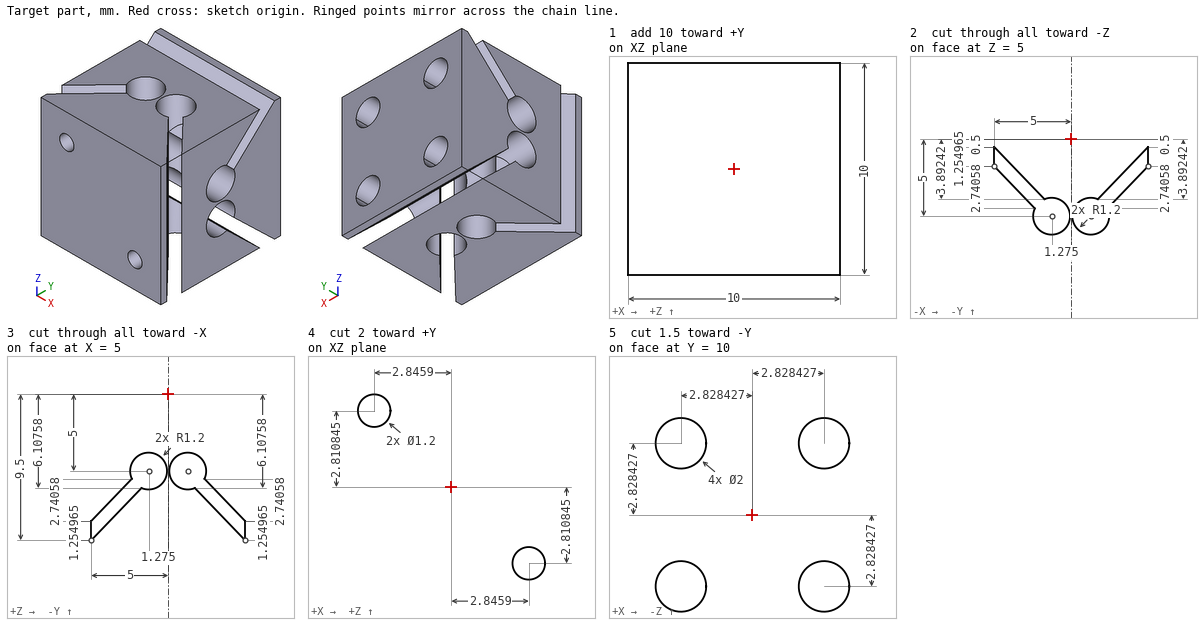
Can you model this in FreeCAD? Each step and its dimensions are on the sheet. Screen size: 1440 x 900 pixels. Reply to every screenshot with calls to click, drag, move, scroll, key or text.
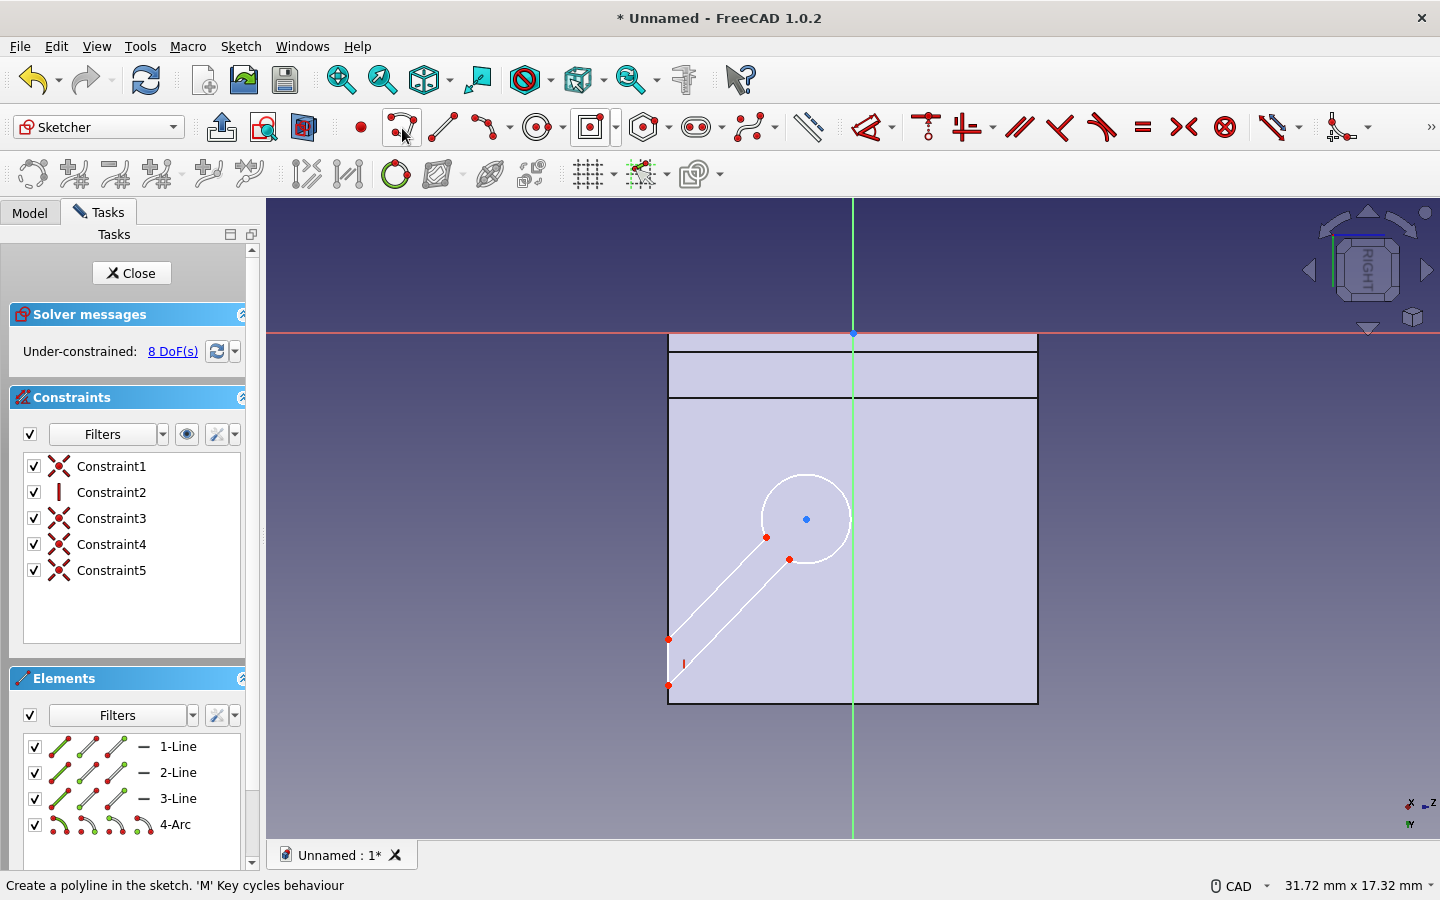
click(917, 559)
click(1038, 685)
click(1038, 639)
click(940, 537)
right_click(940, 537)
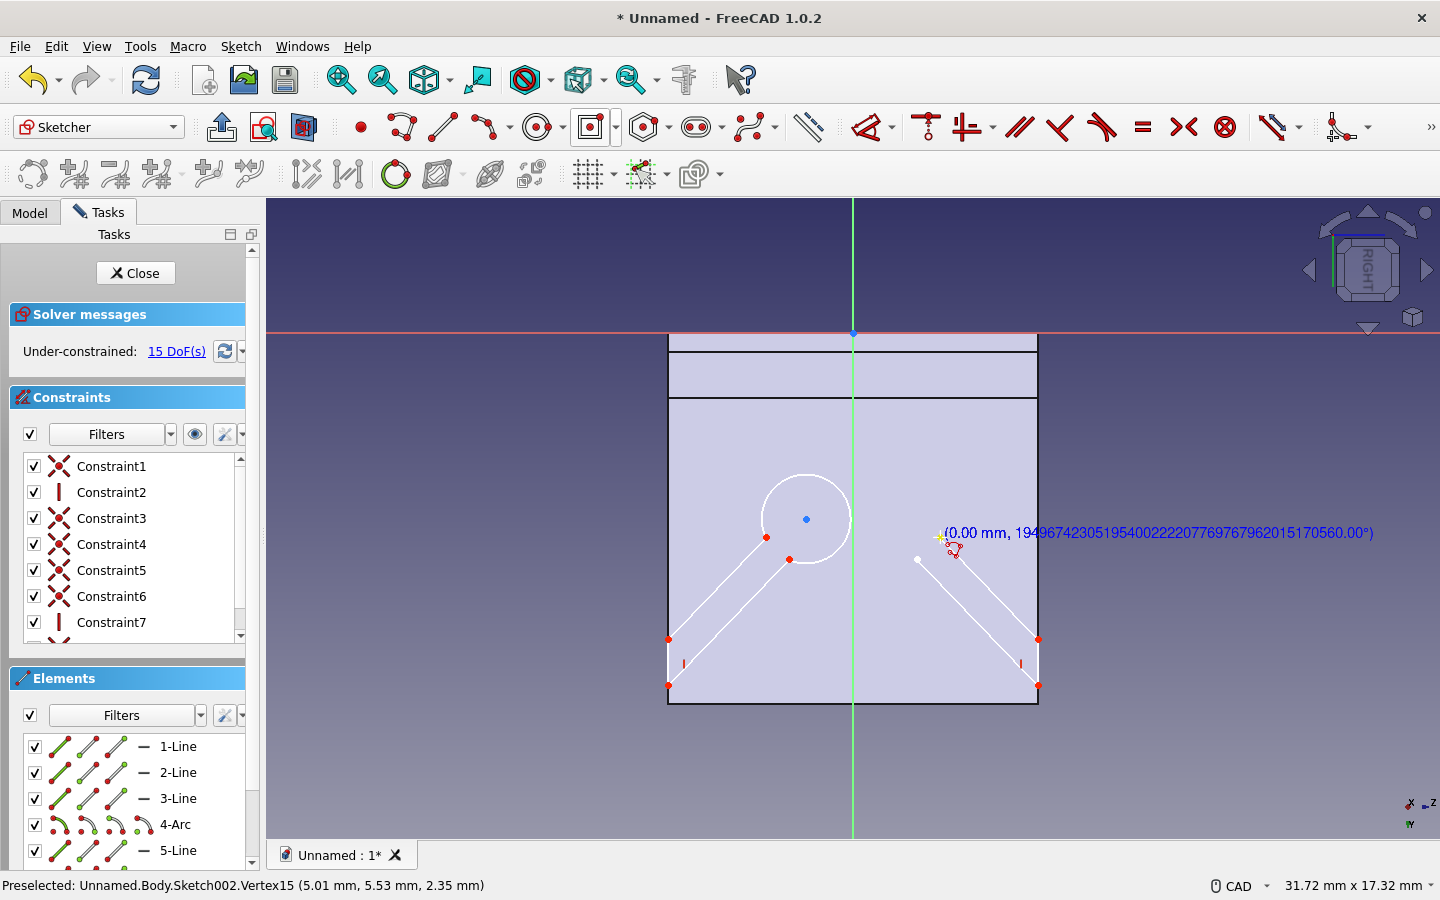
key(g)
key(3)
key(a)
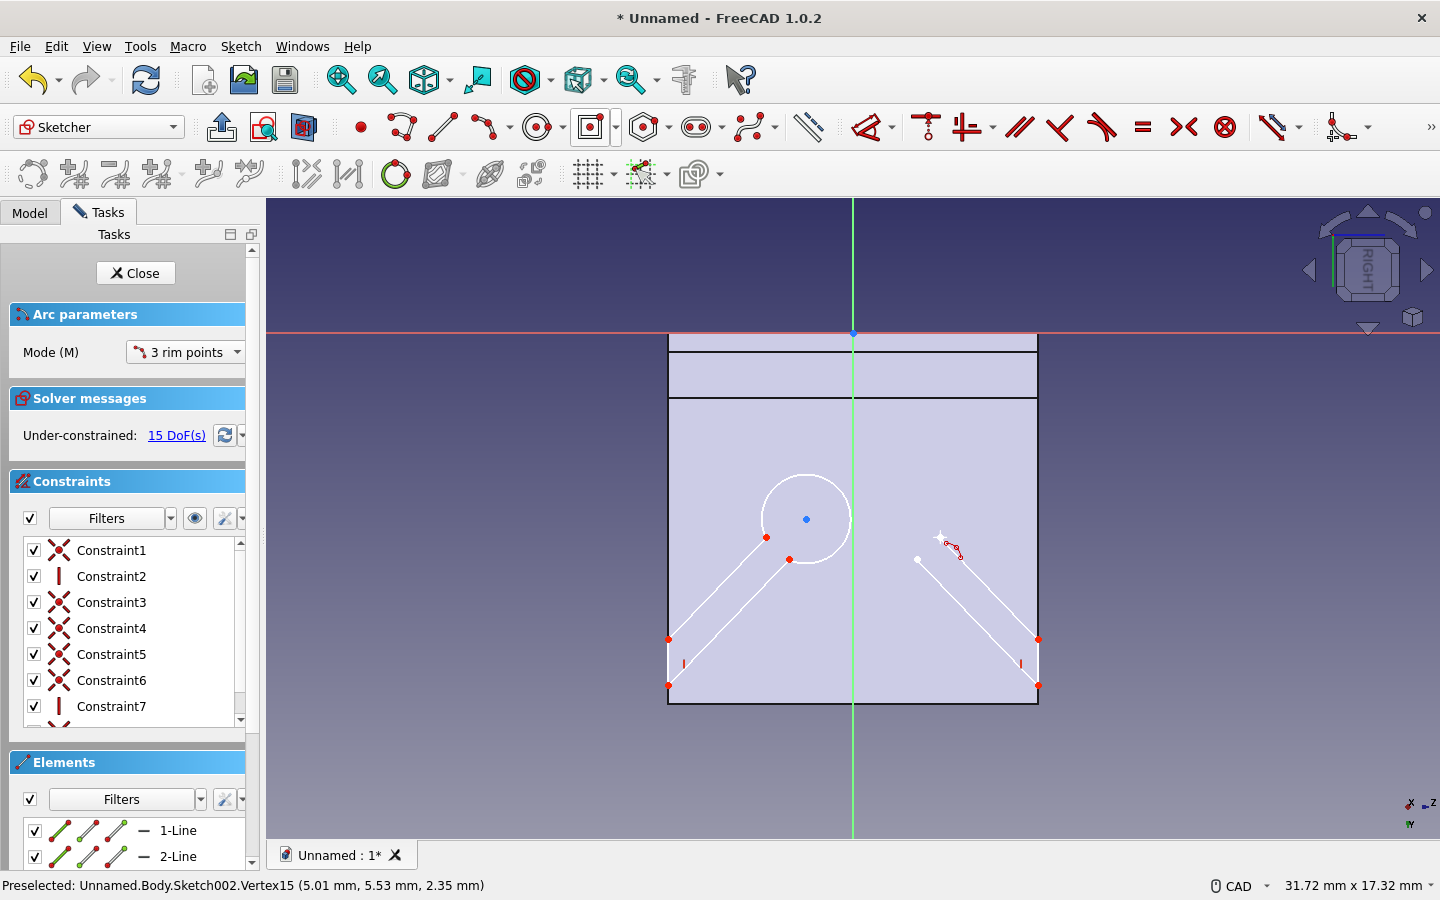
click(940, 538)
click(917, 560)
click(869, 486)
key(Escape)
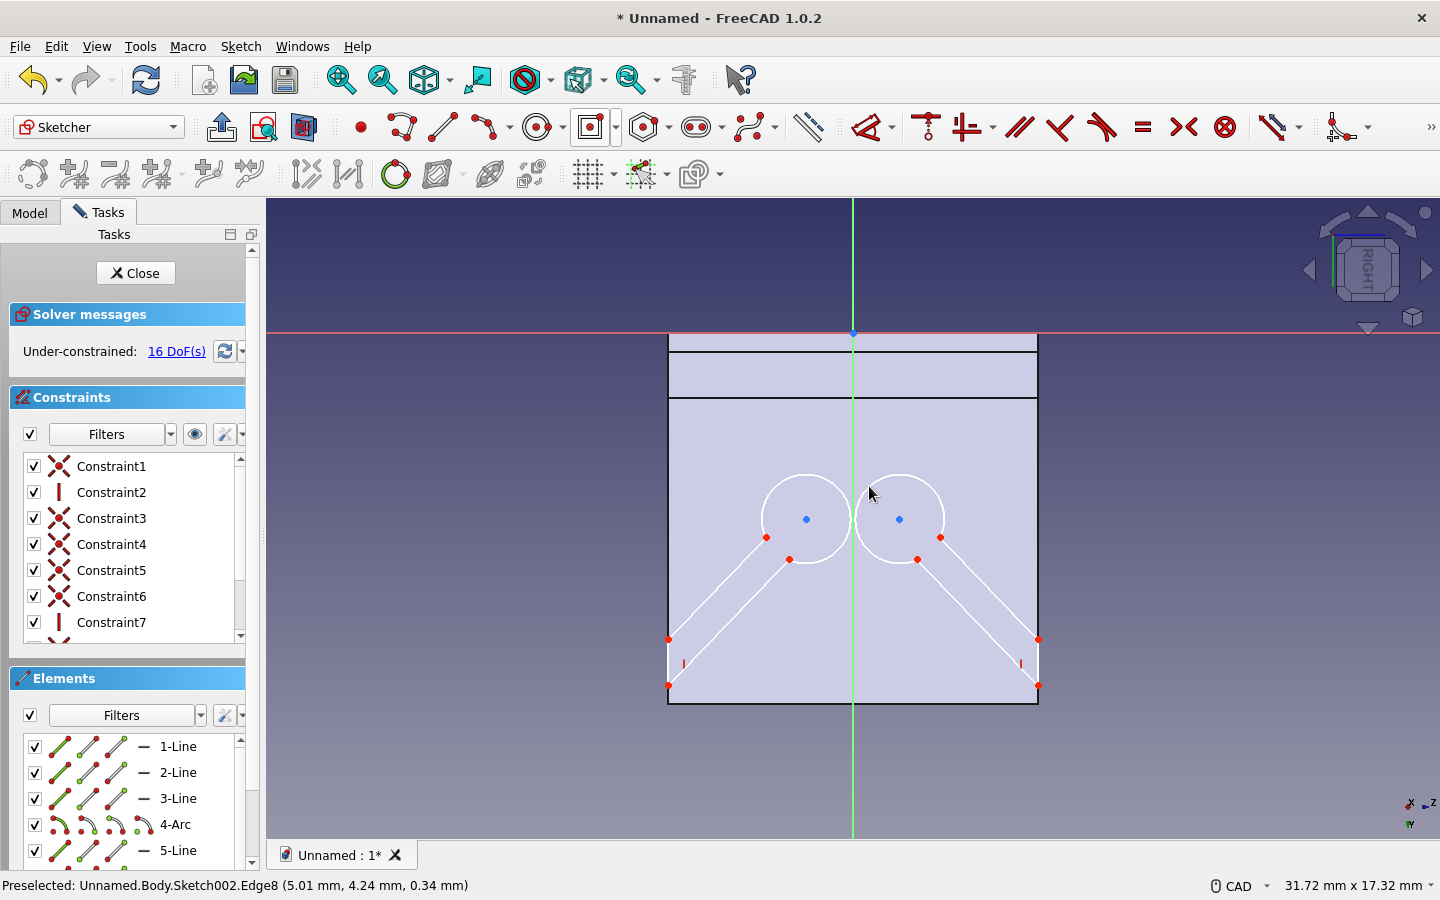
click(791, 477)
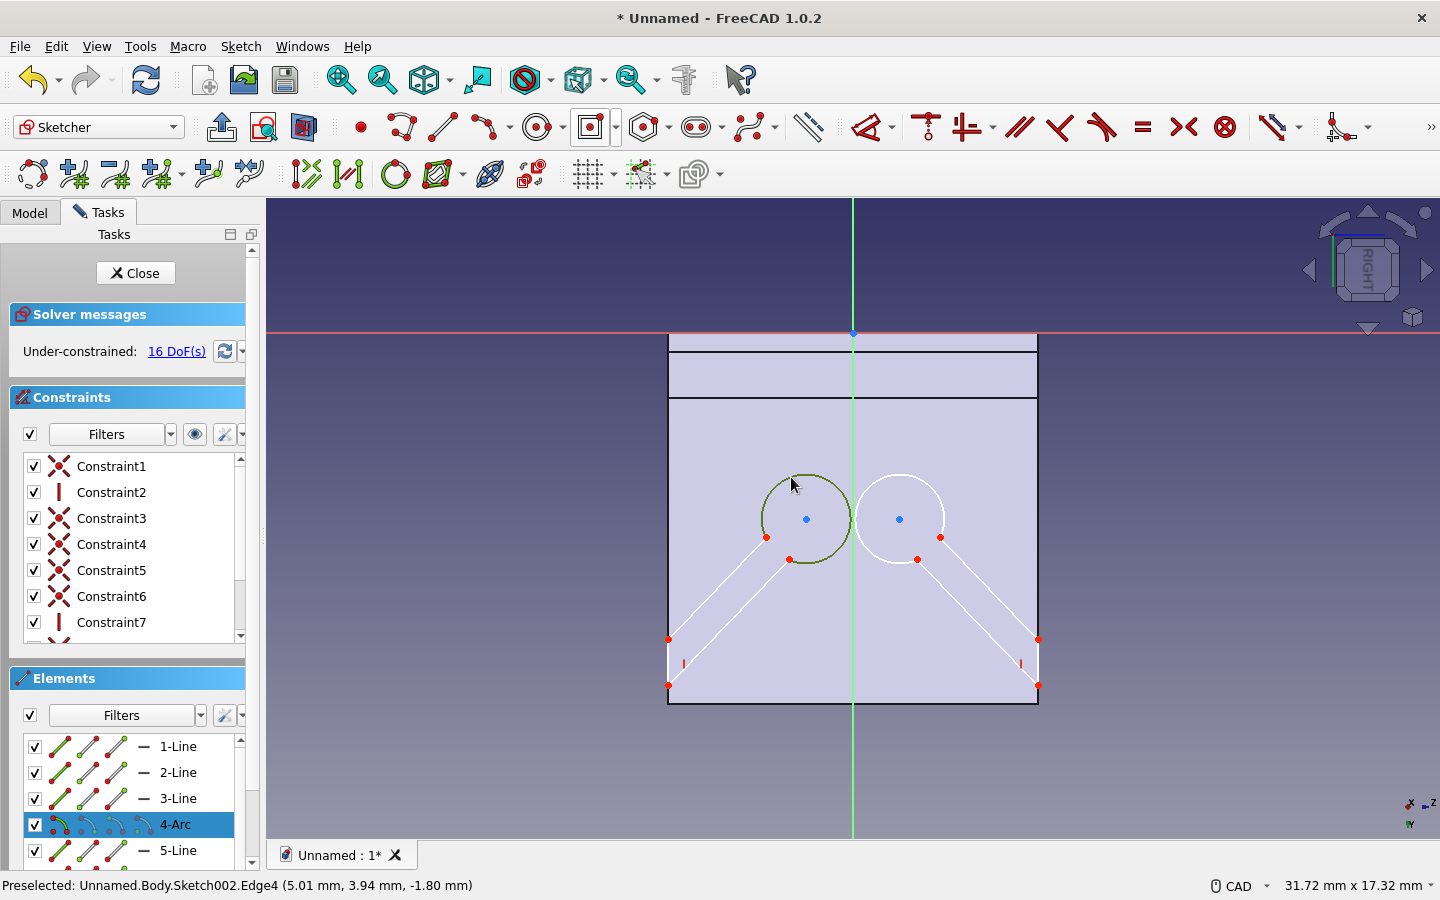
click(915, 477)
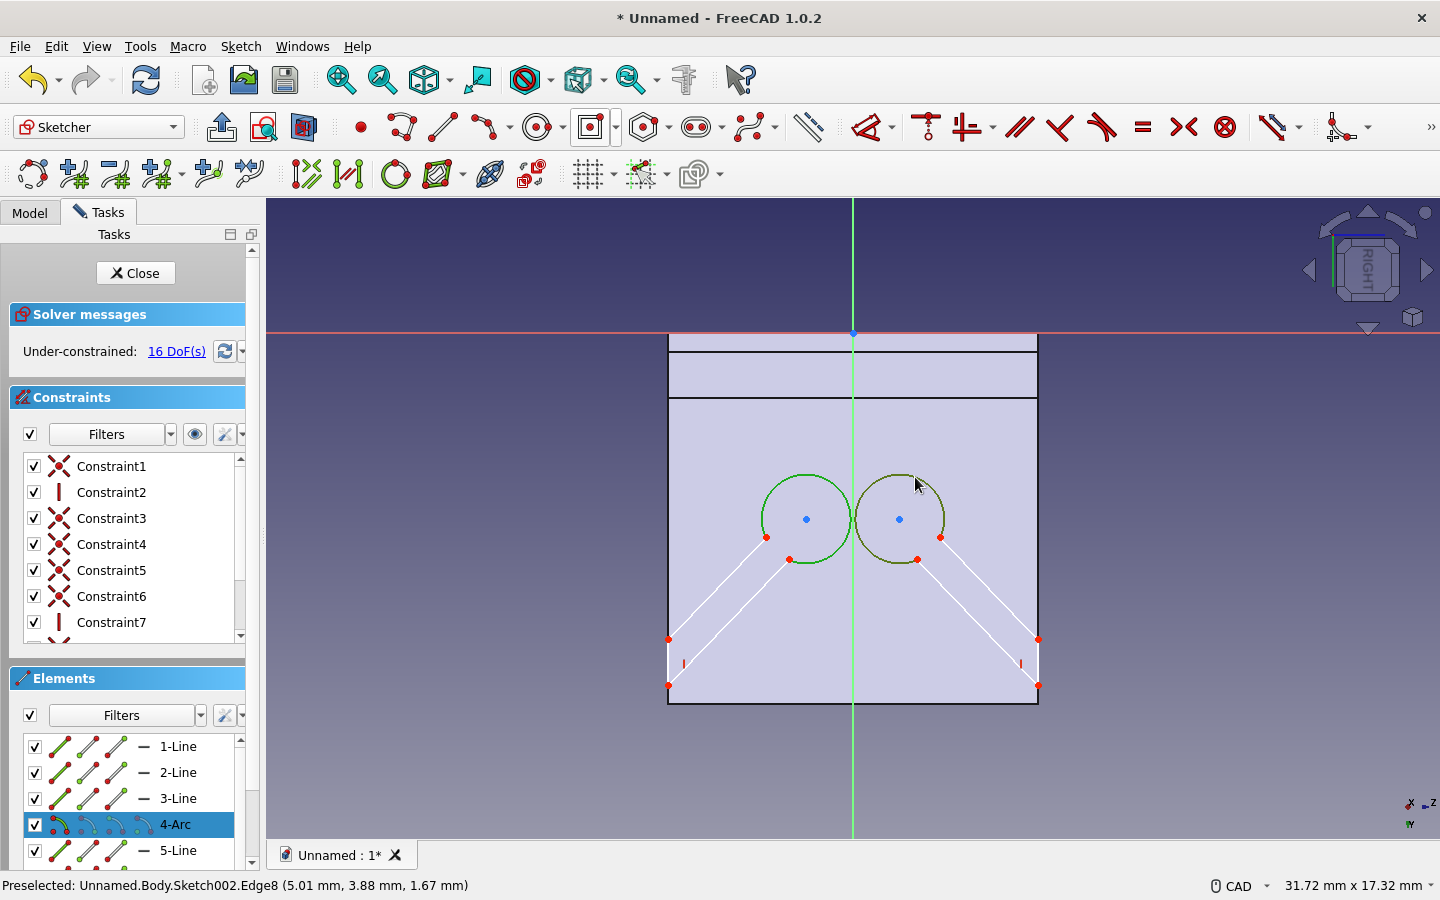
click(1143, 128)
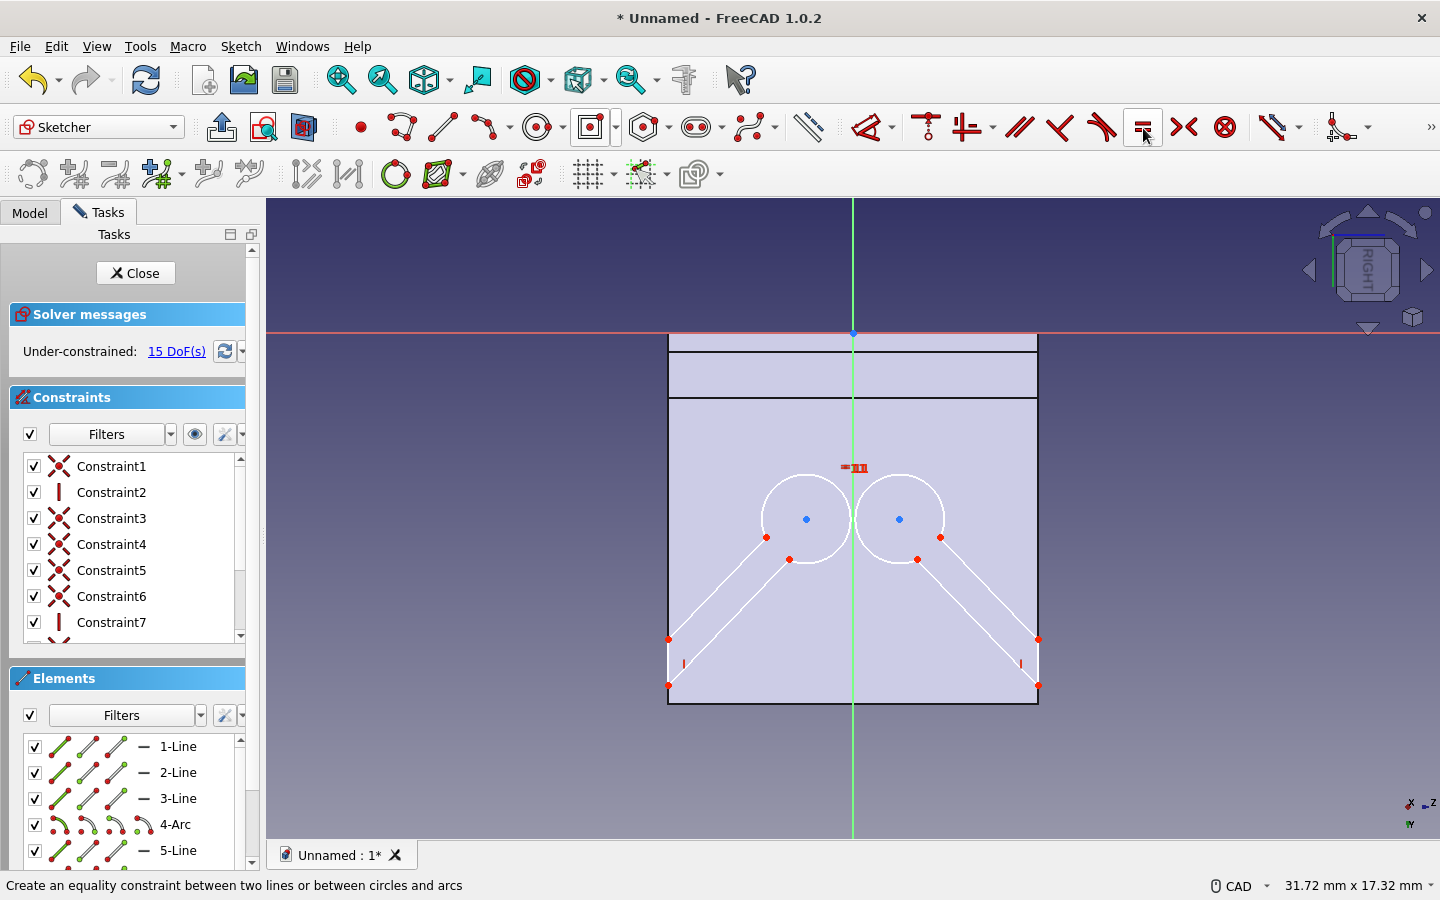
click(806, 519)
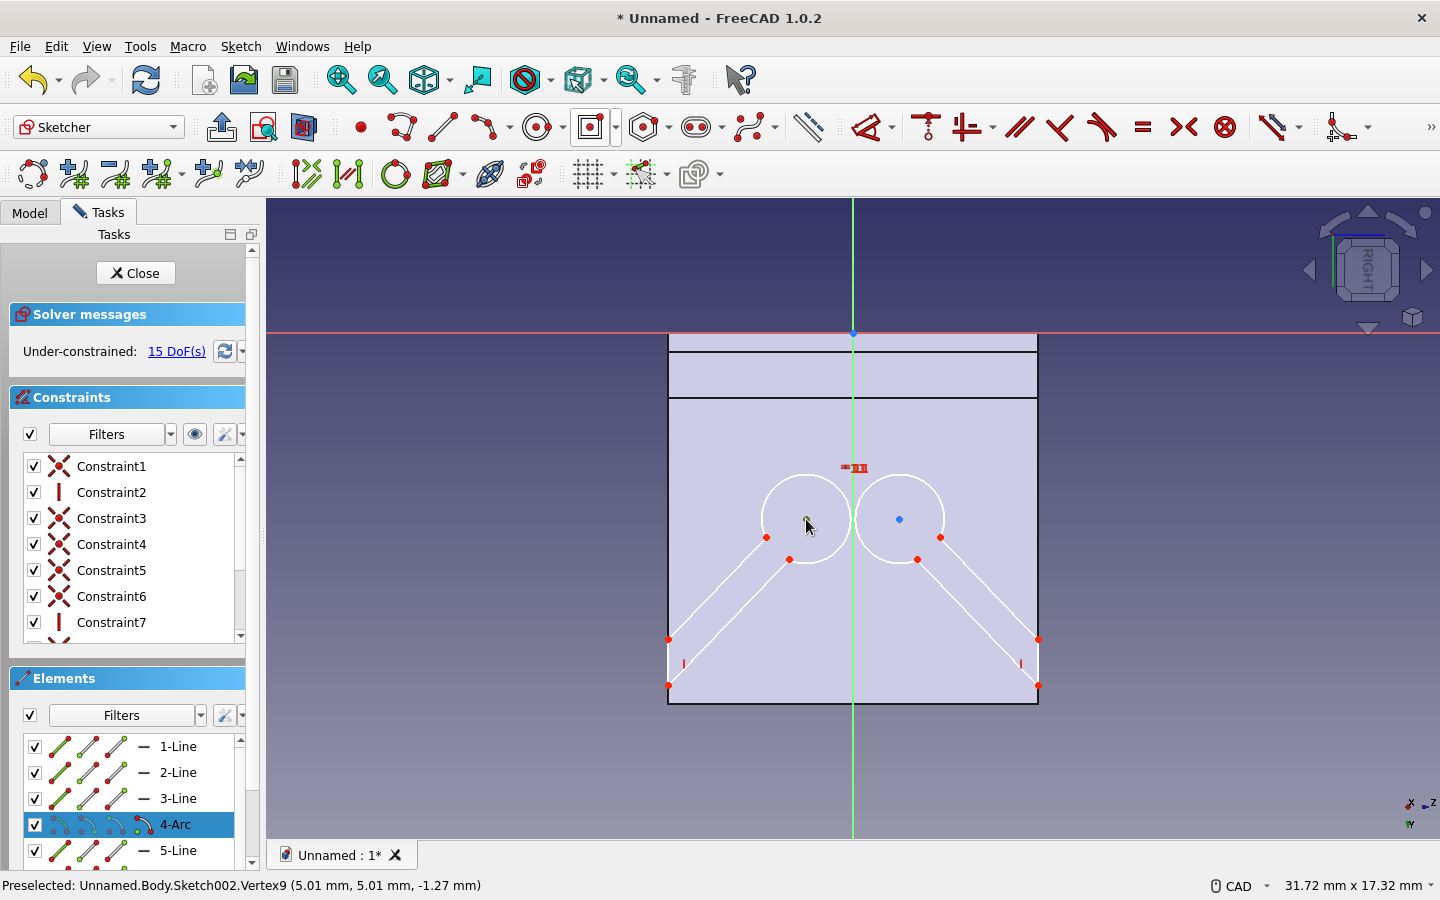
click(900, 519)